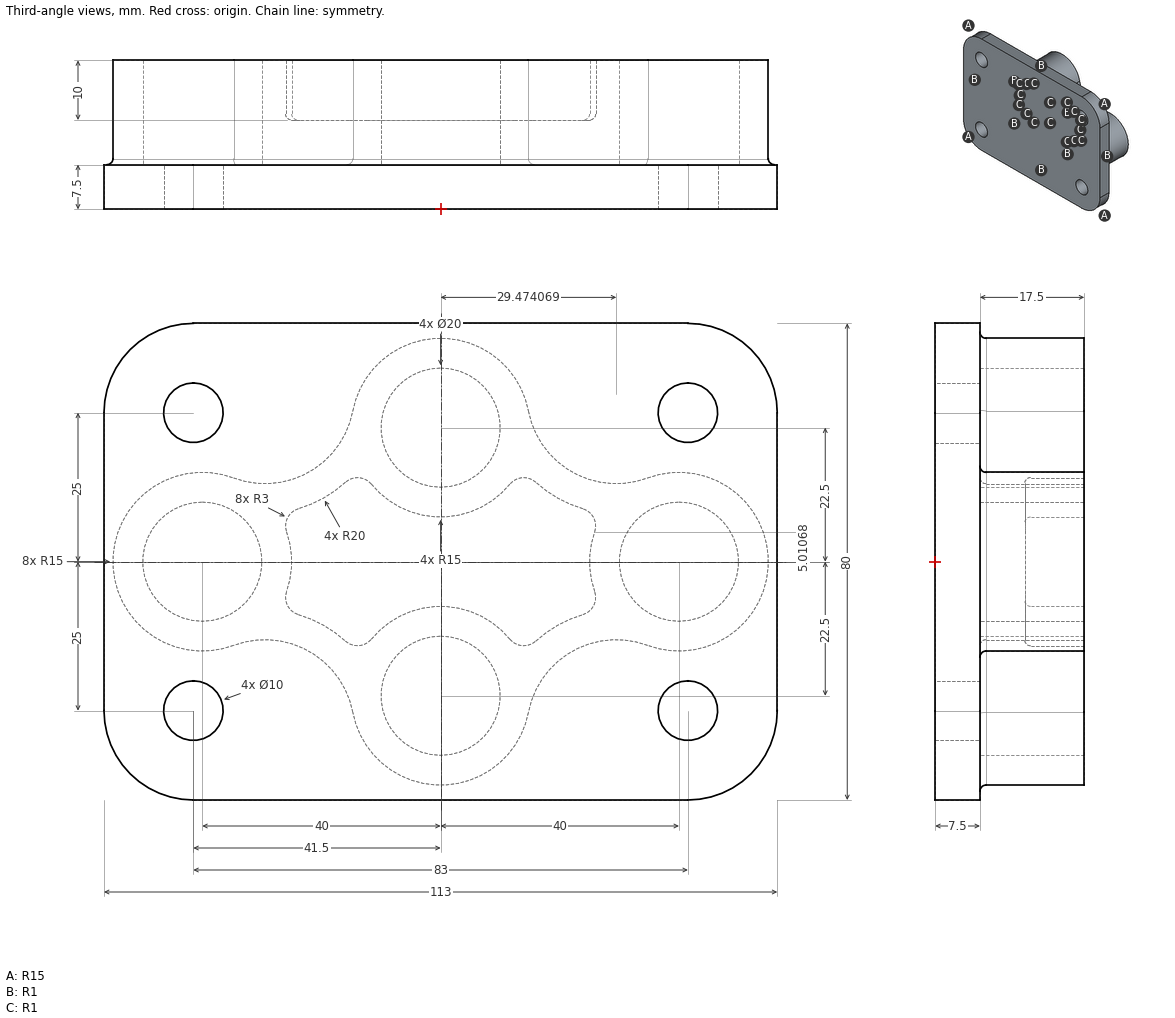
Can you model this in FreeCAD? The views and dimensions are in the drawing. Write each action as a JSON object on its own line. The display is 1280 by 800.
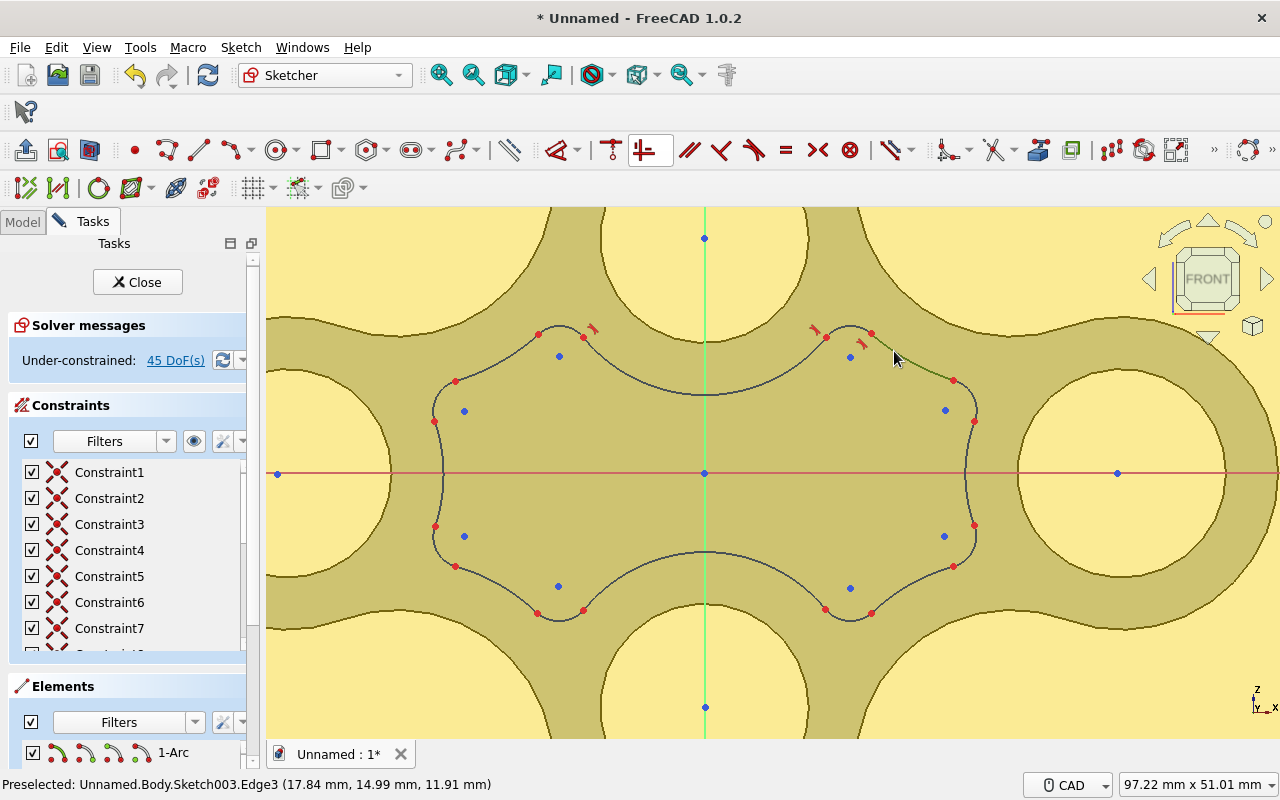
{"action": "left_click", "coordinate": [976, 406]}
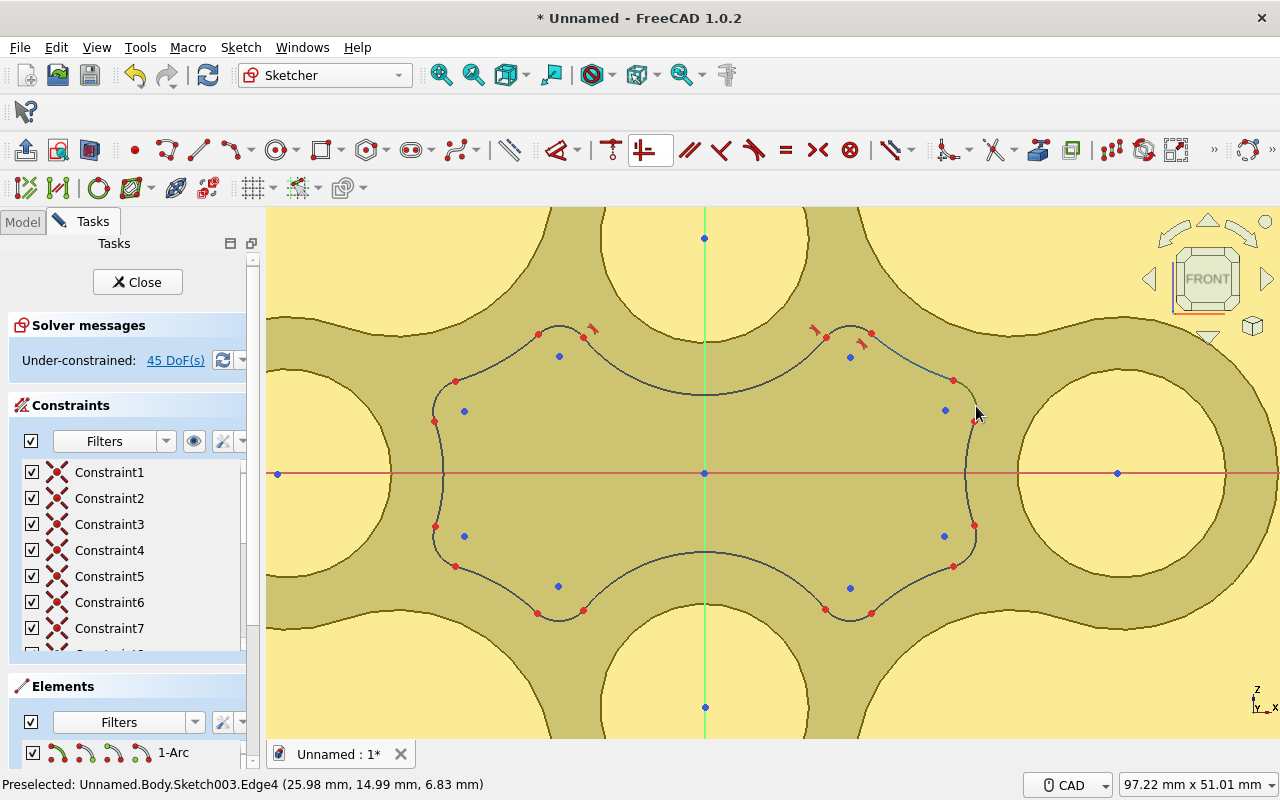
{"action": "key", "text": "t"}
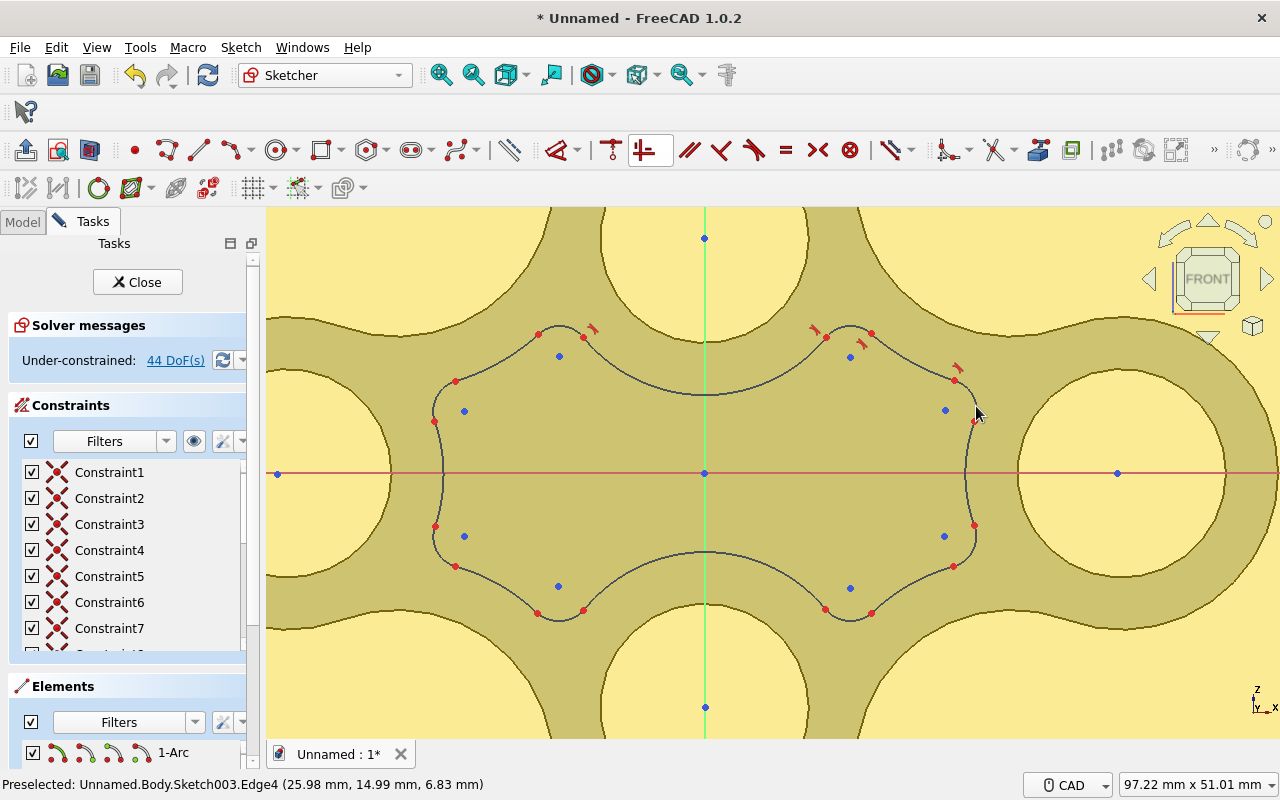
{"action": "left_click", "coordinate": [976, 407]}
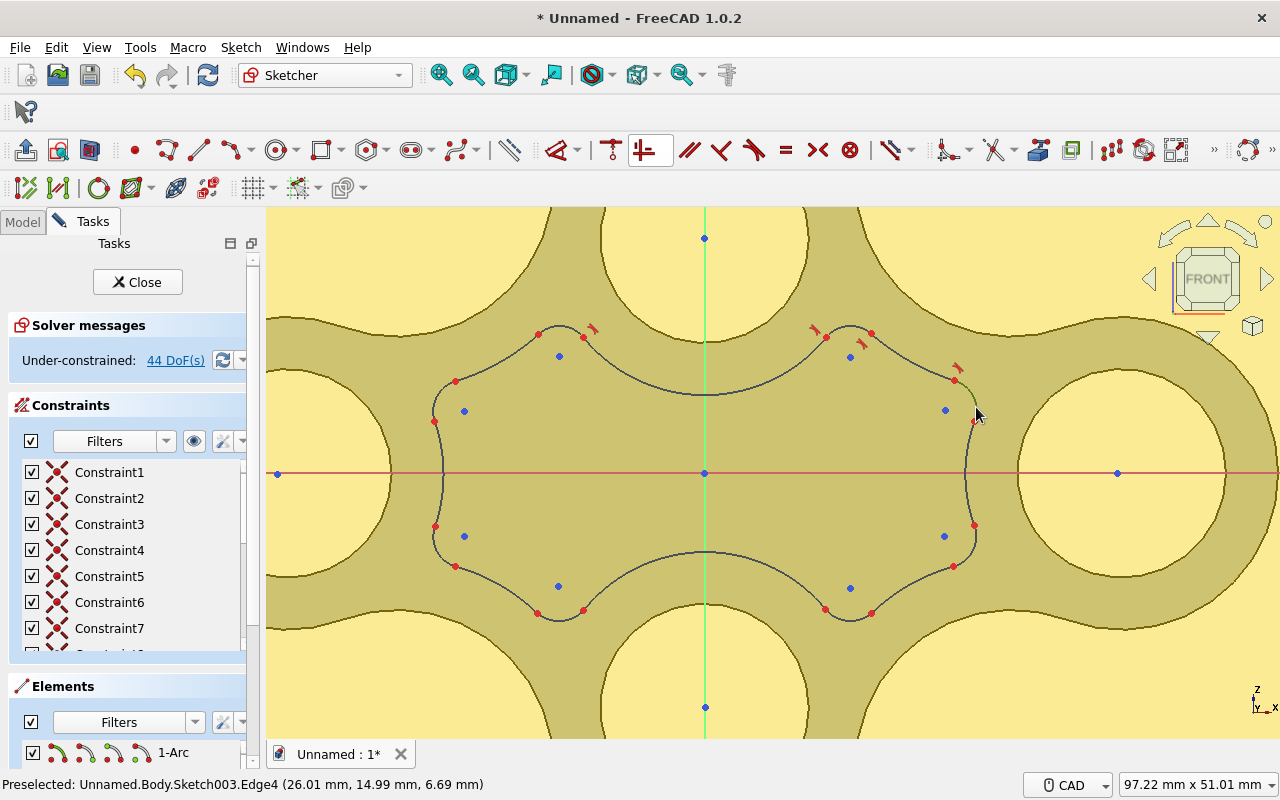
{"action": "left_click", "coordinate": [967, 453]}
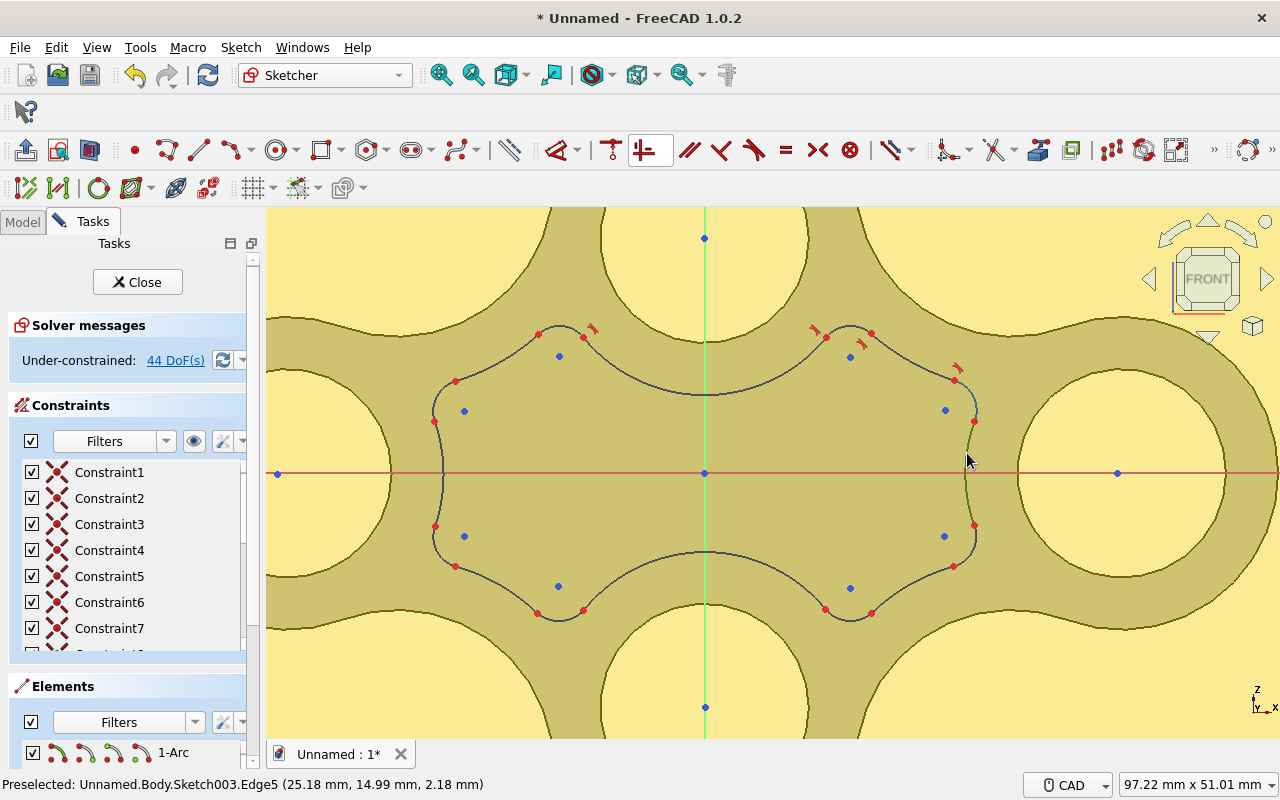
{"action": "left_click", "coordinate": [754, 150]}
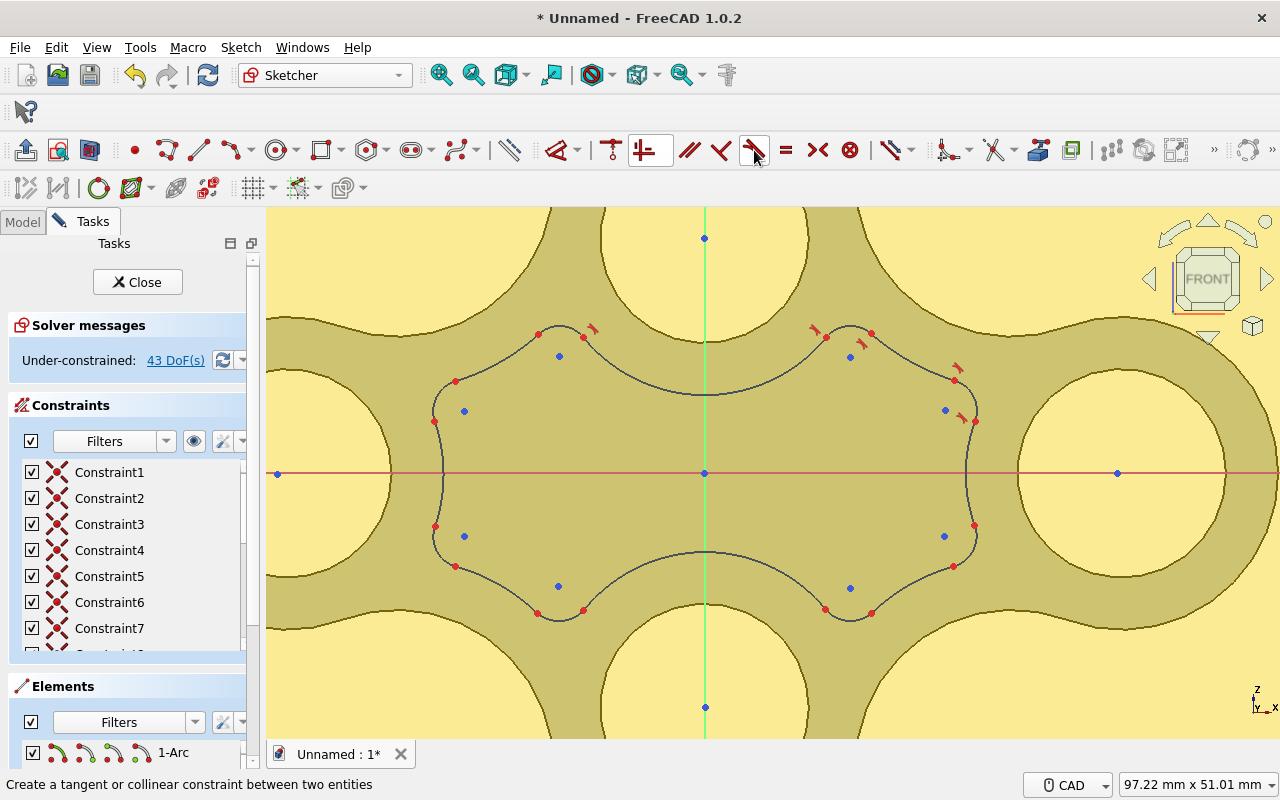
{"action": "left_click", "coordinate": [967, 453]}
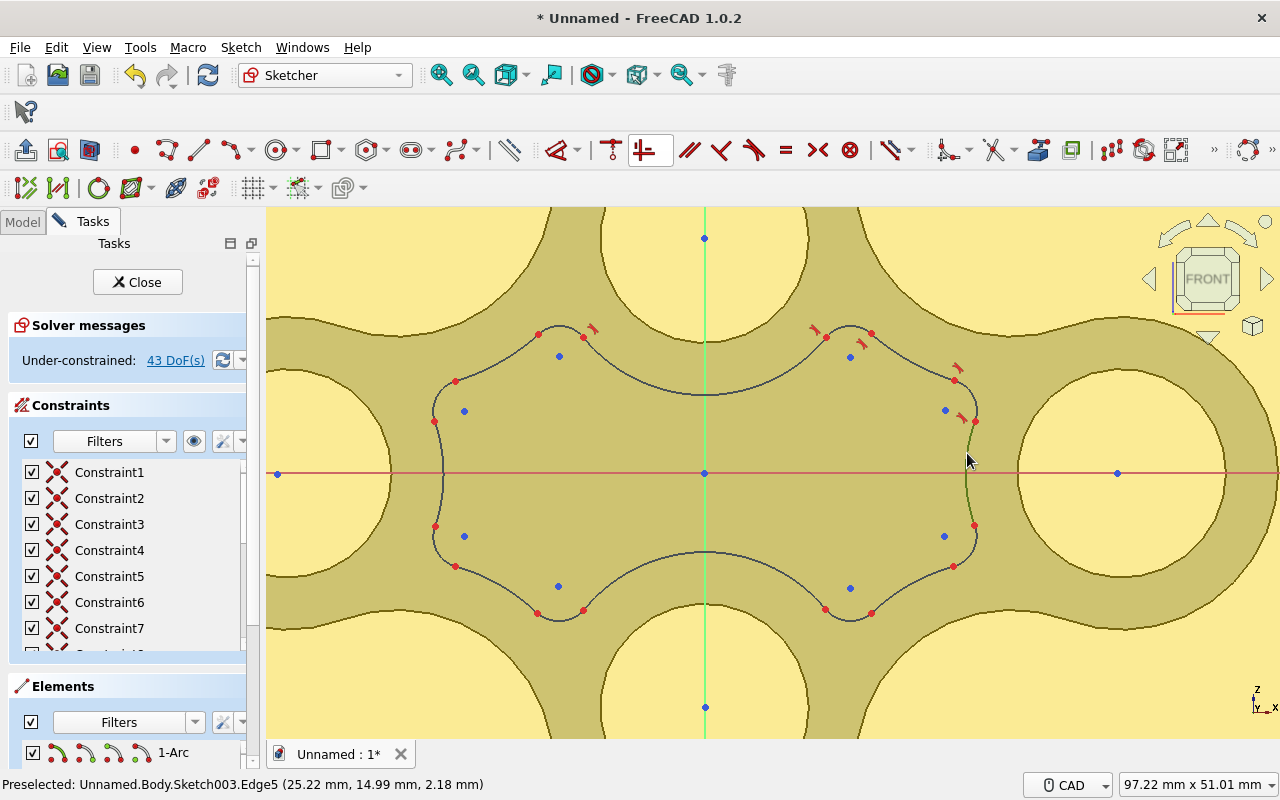
{"action": "left_click", "coordinate": [967, 559]}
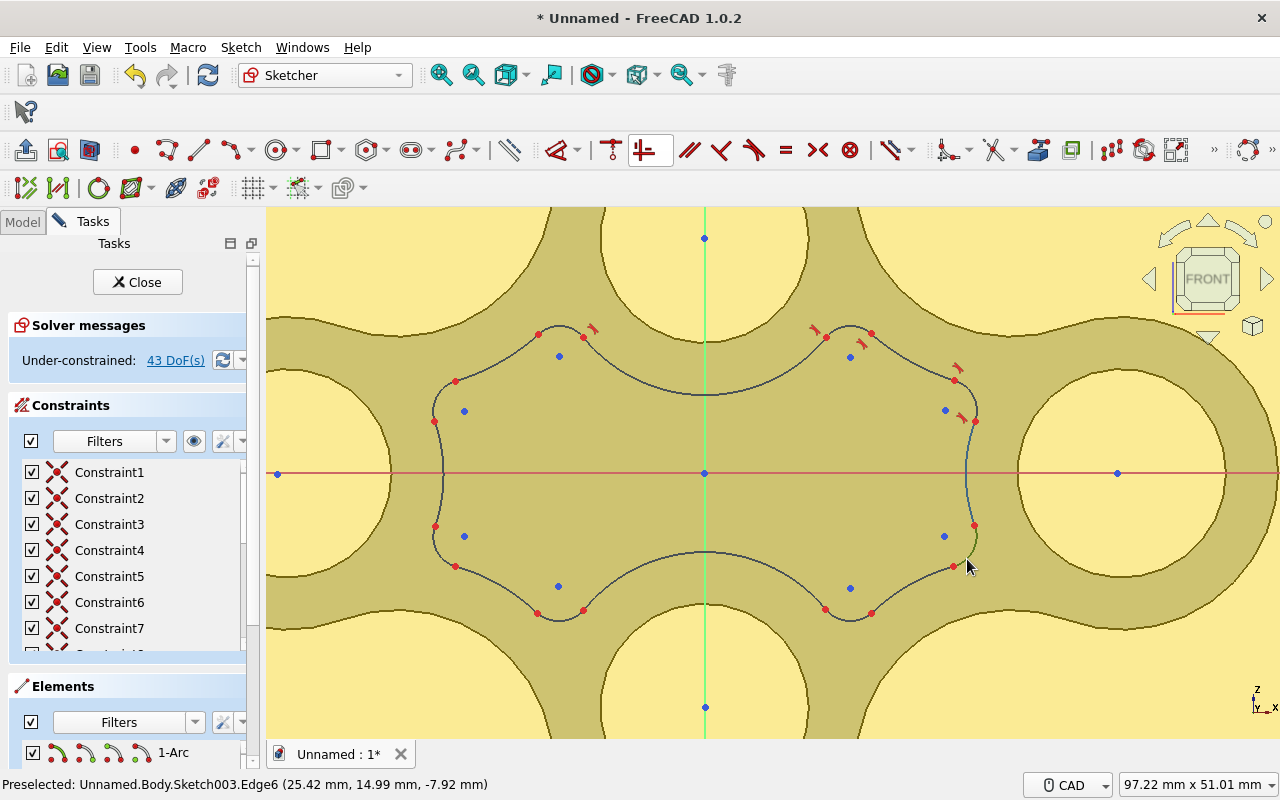
{"action": "left_click", "coordinate": [754, 150]}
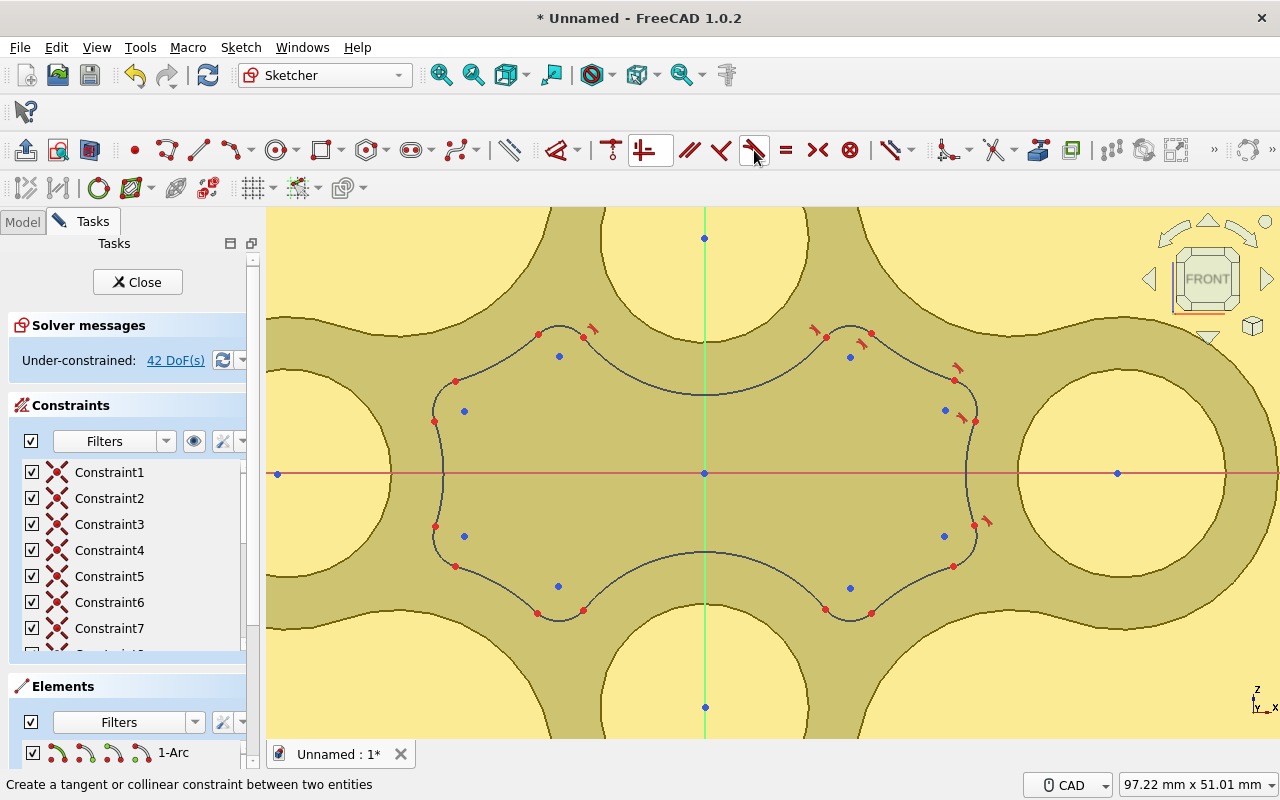
{"action": "left_click", "coordinate": [967, 559]}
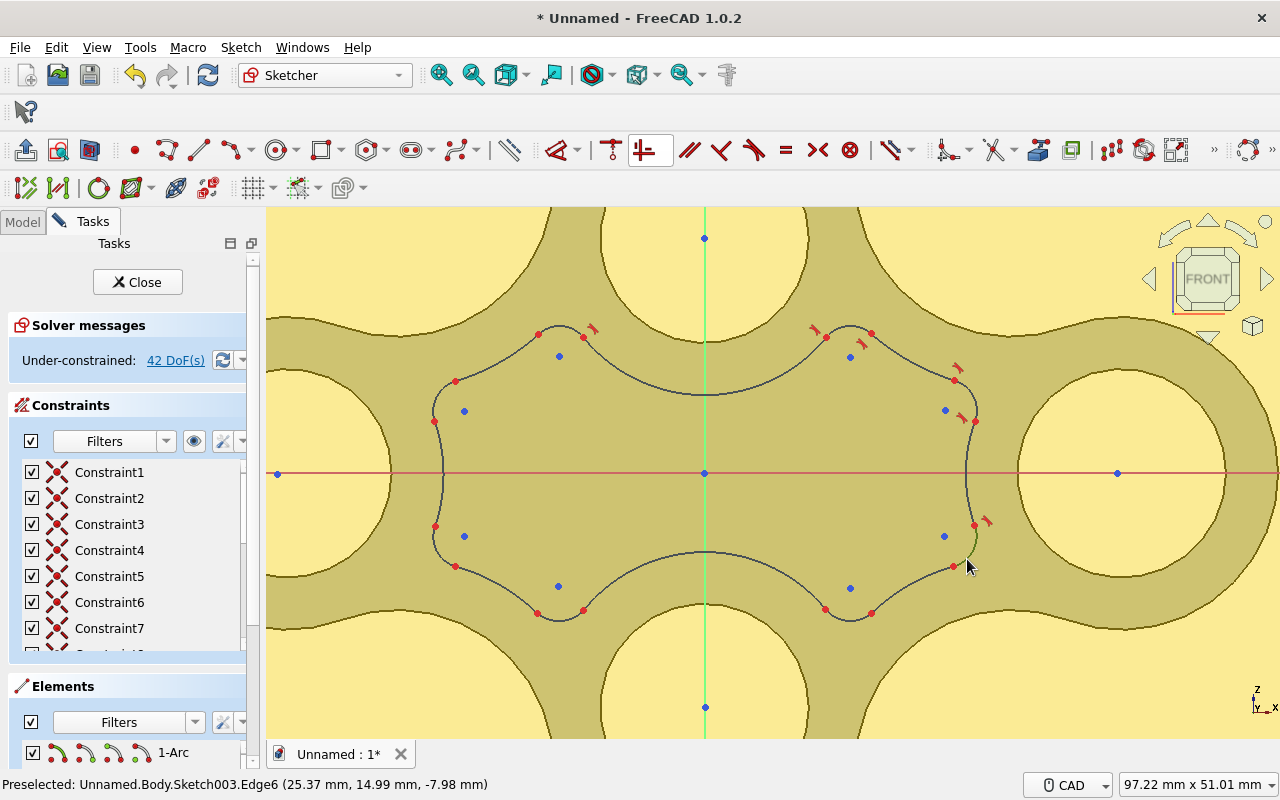
{"action": "left_click", "coordinate": [927, 576]}